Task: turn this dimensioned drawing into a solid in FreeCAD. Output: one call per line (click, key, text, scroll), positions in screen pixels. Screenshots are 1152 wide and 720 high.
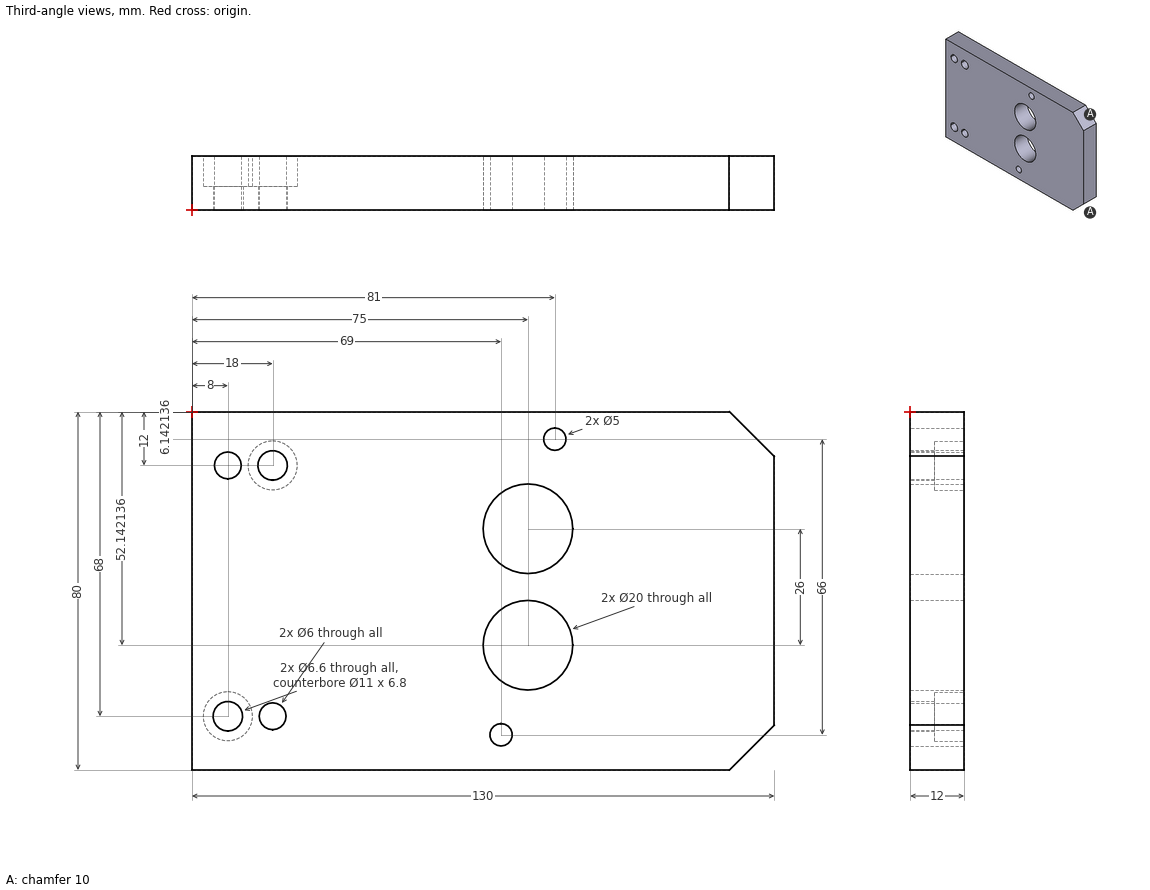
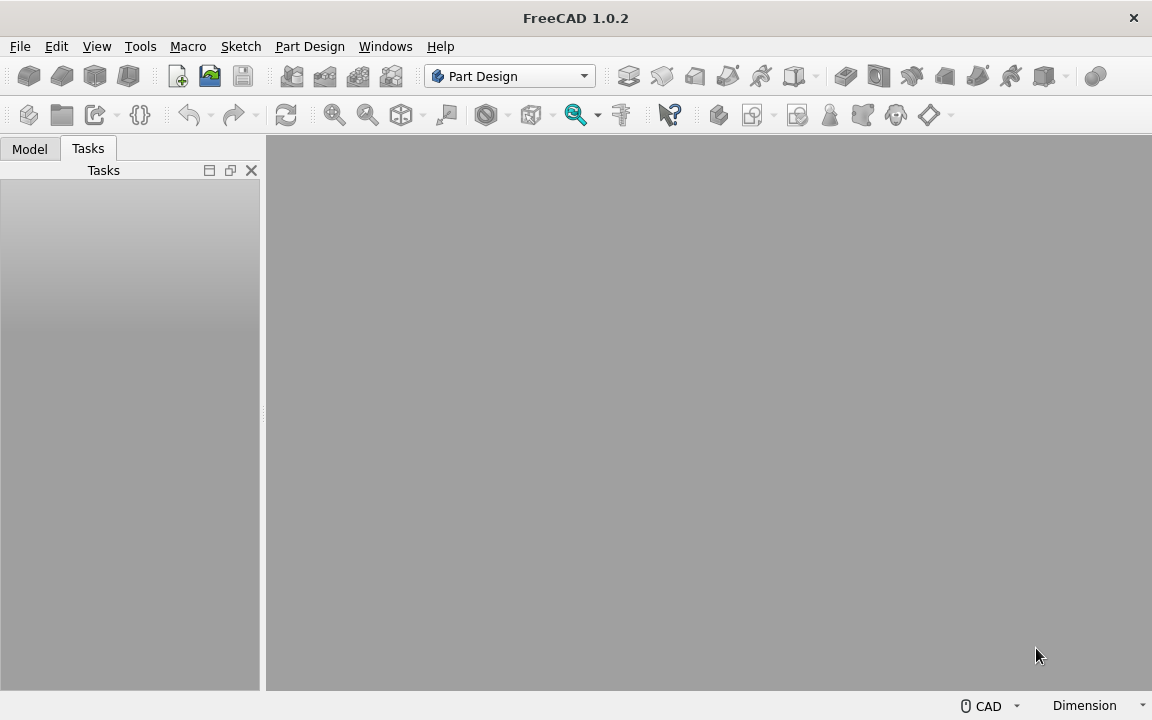
key(ctrl+n)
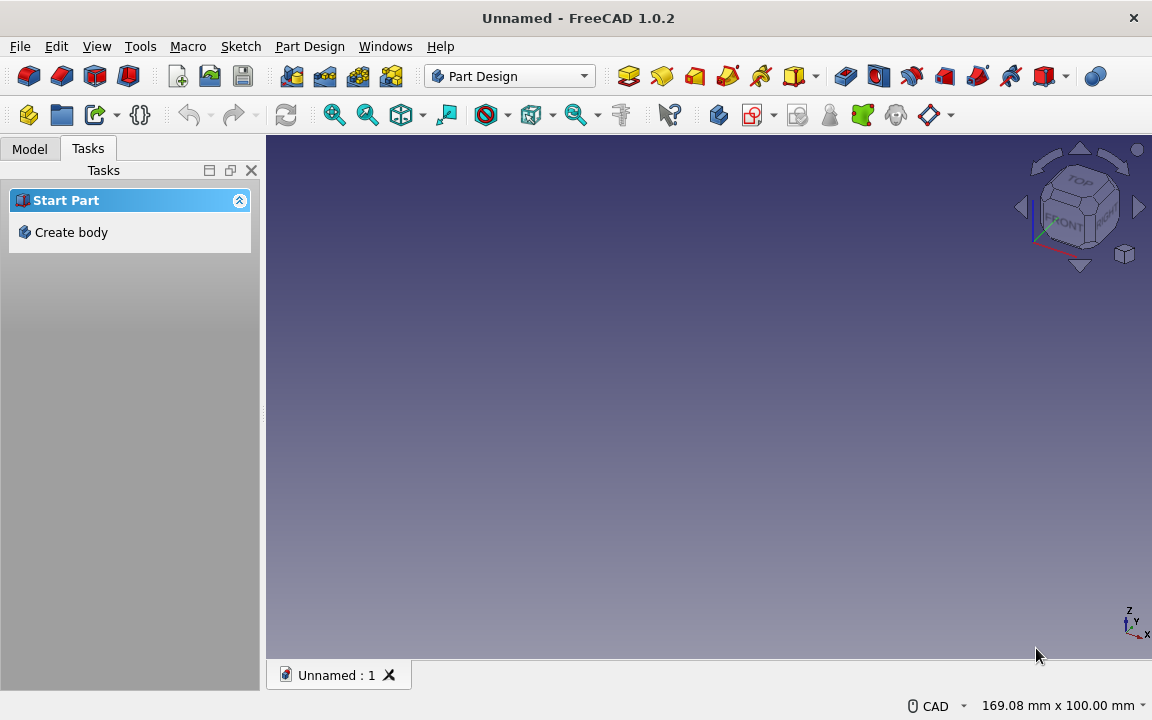
click(752, 116)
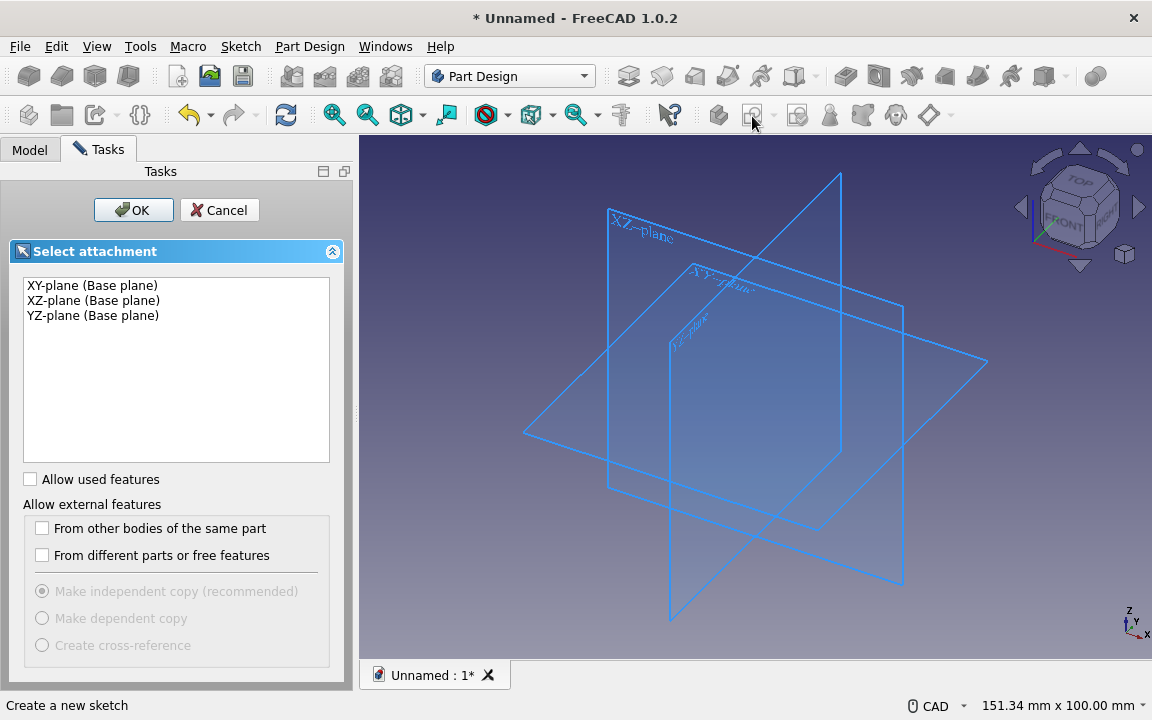
click(84, 300)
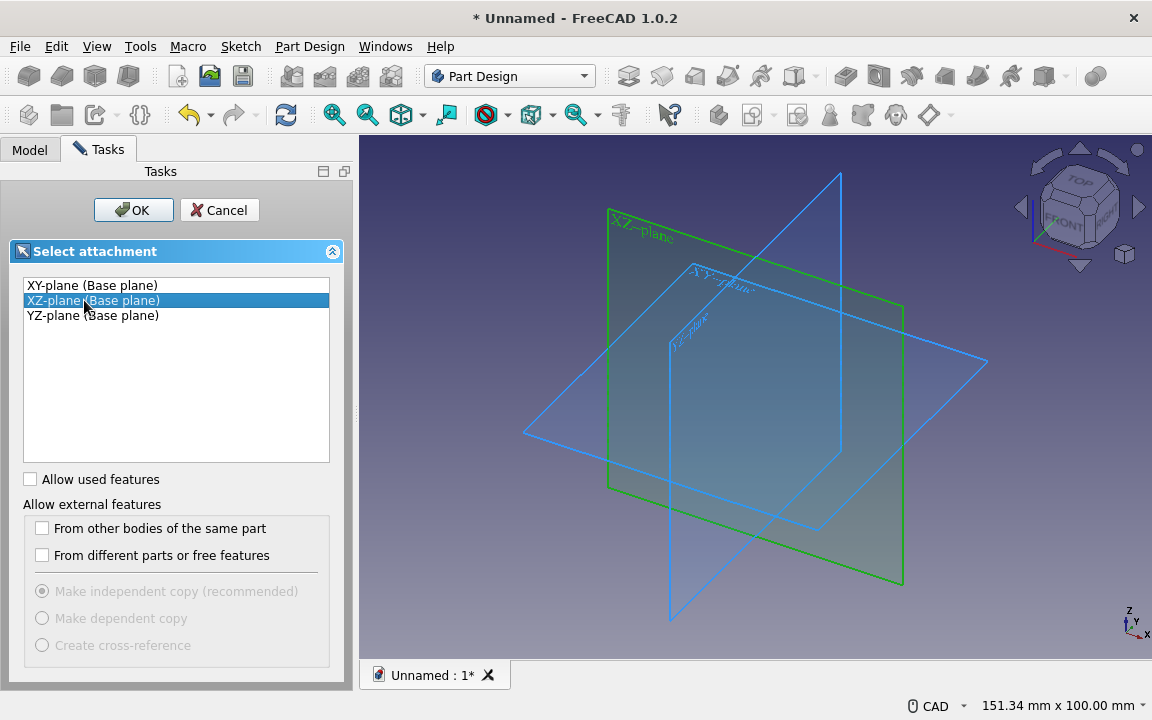
click(134, 210)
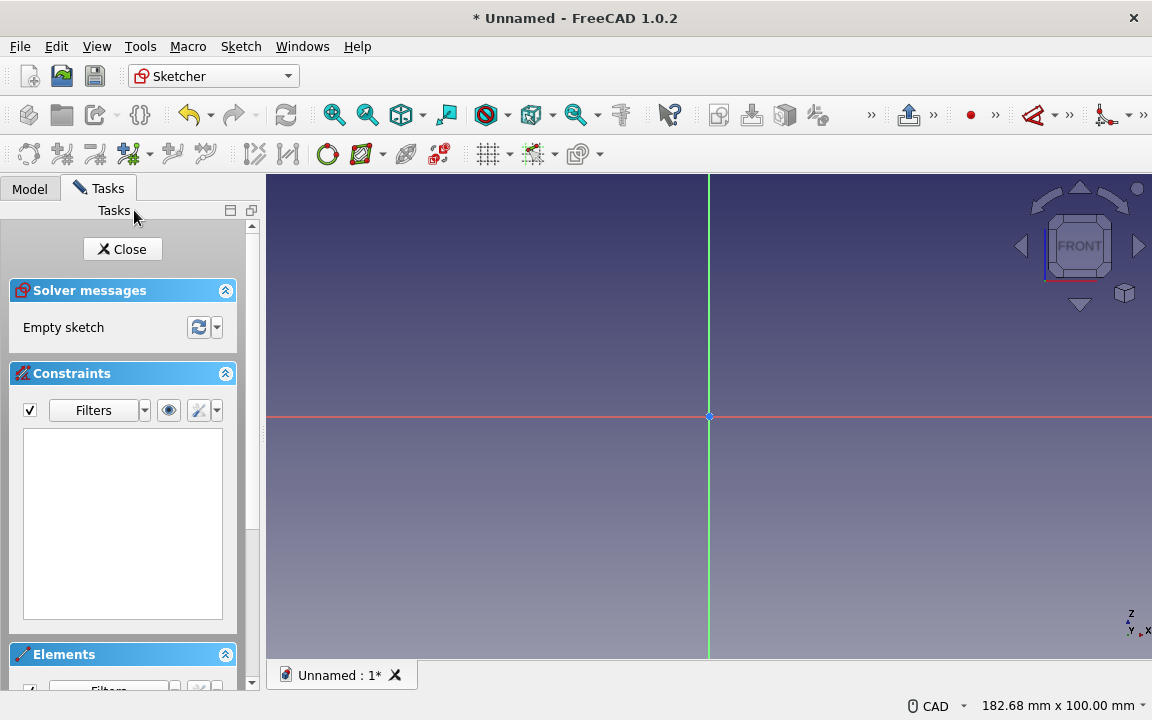
scroll(294, 202, down, 3)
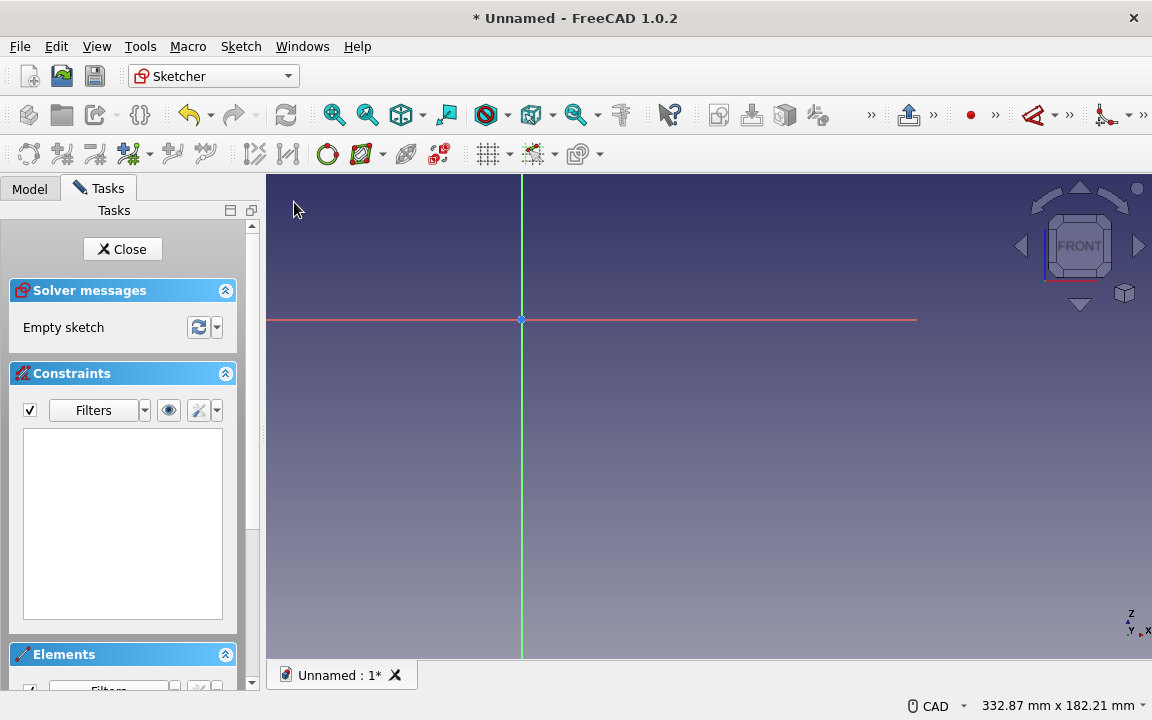
scroll(805, 446, up, 2)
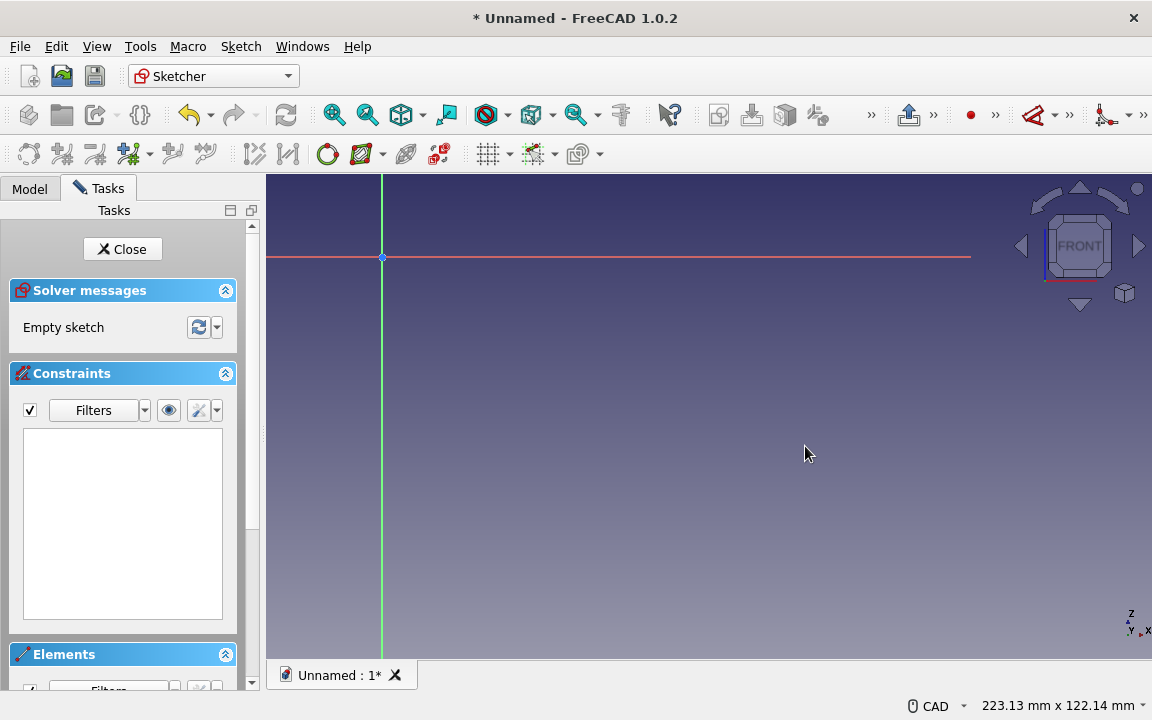
key(g)
key(r)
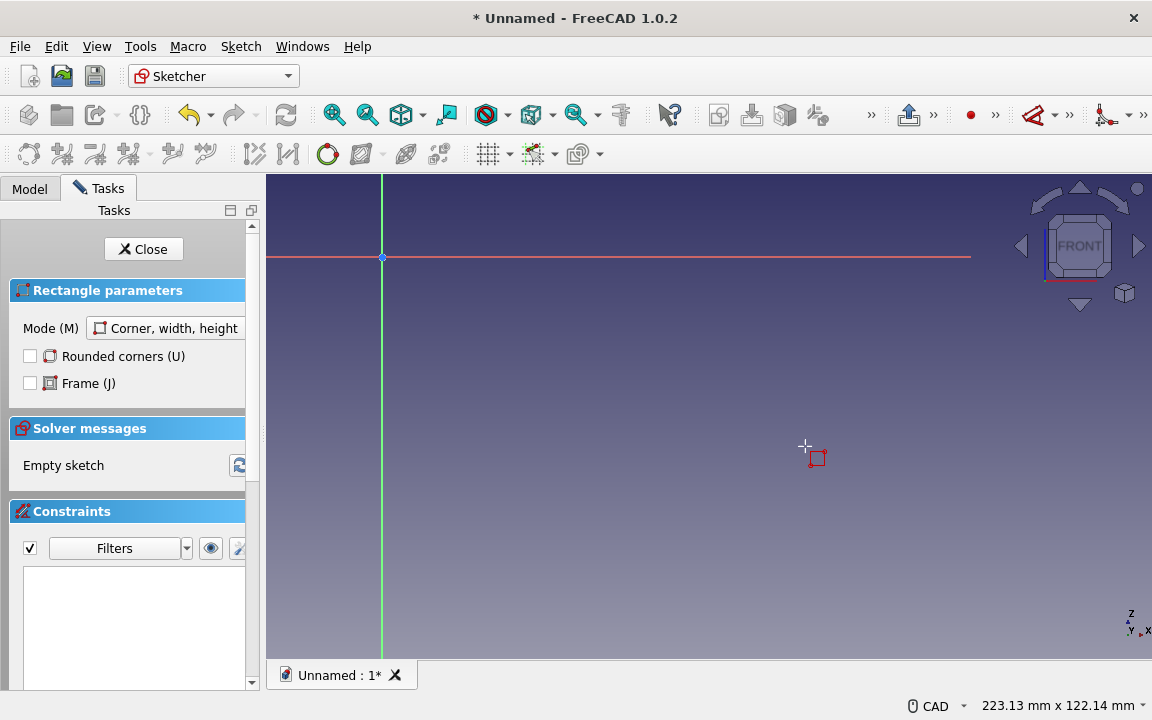
click(382, 257)
click(898, 575)
key(Escape)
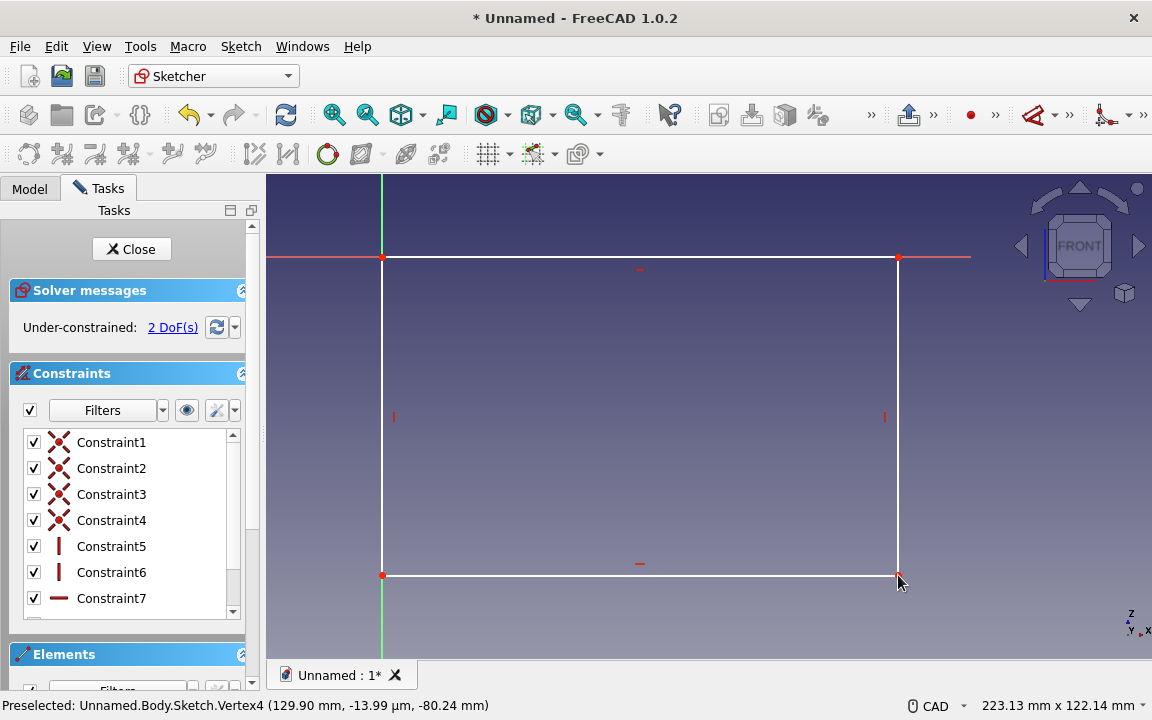
key(d)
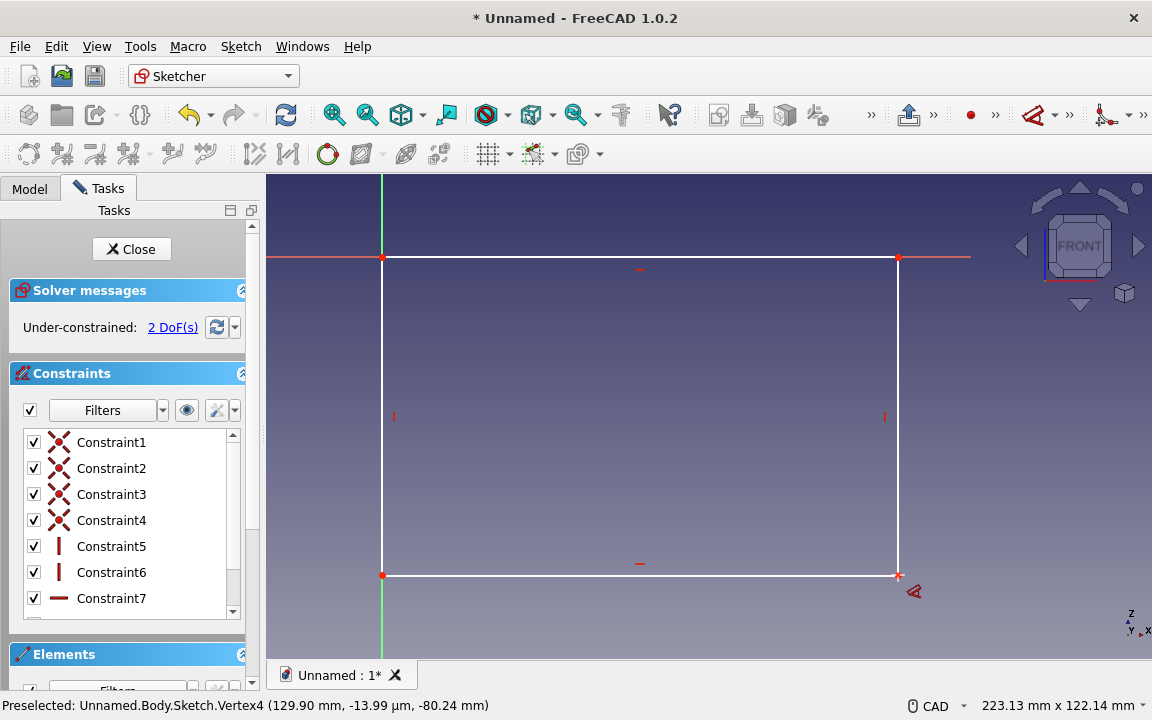
click(382, 353)
click(348, 417)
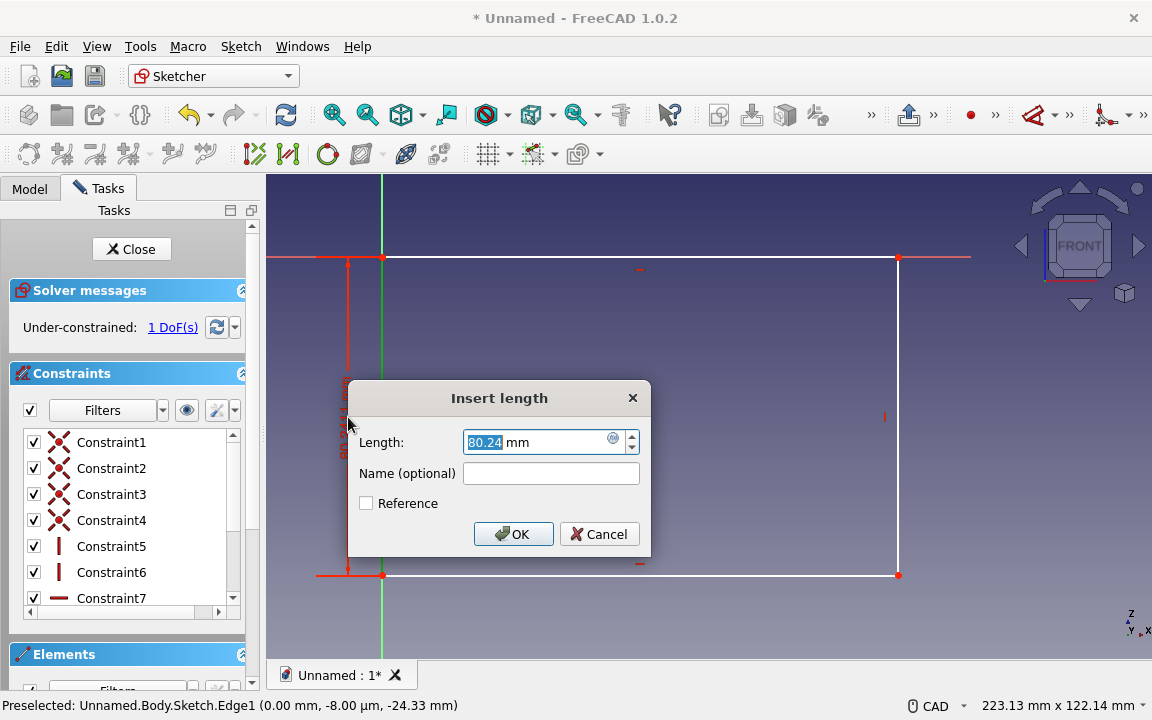
text(80)
key(Return)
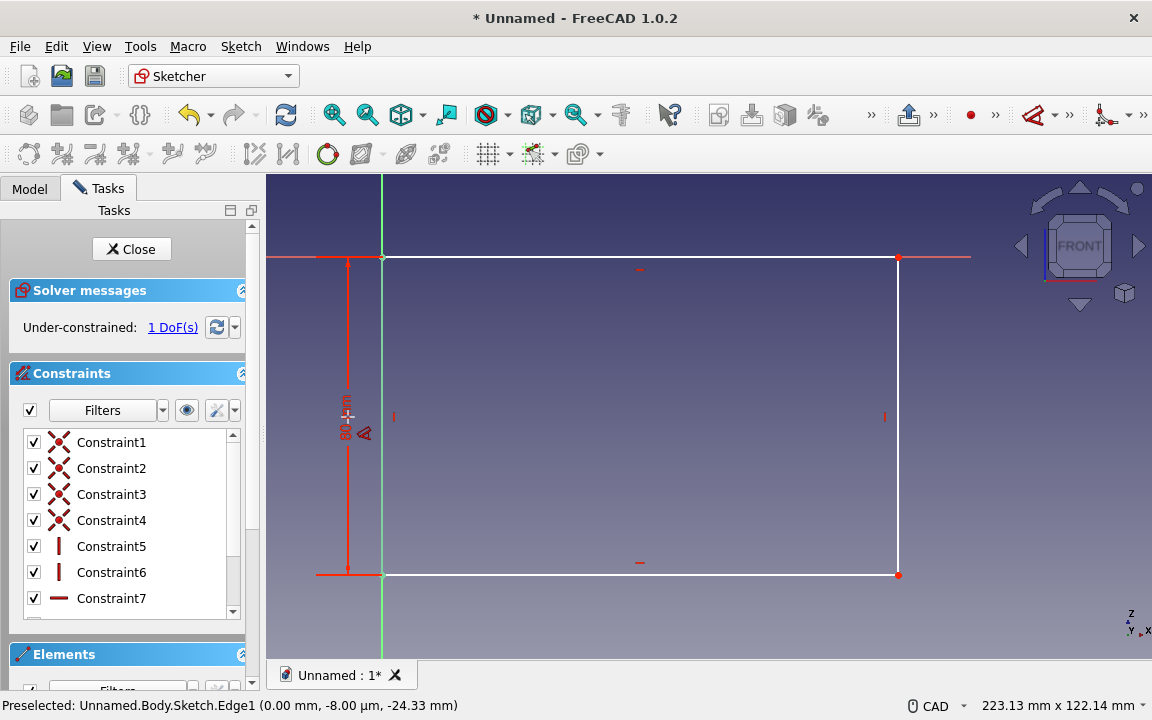
click(537, 575)
click(640, 609)